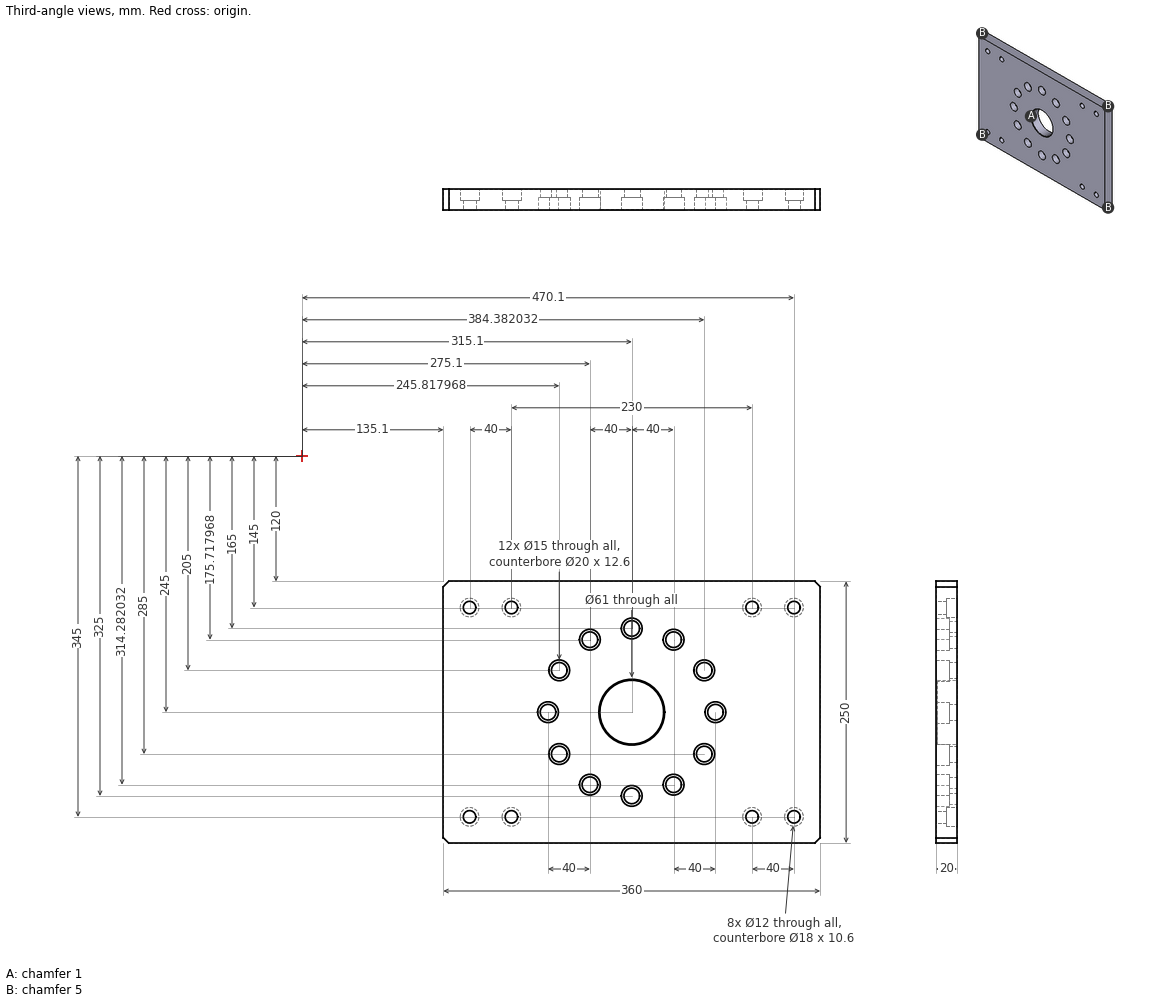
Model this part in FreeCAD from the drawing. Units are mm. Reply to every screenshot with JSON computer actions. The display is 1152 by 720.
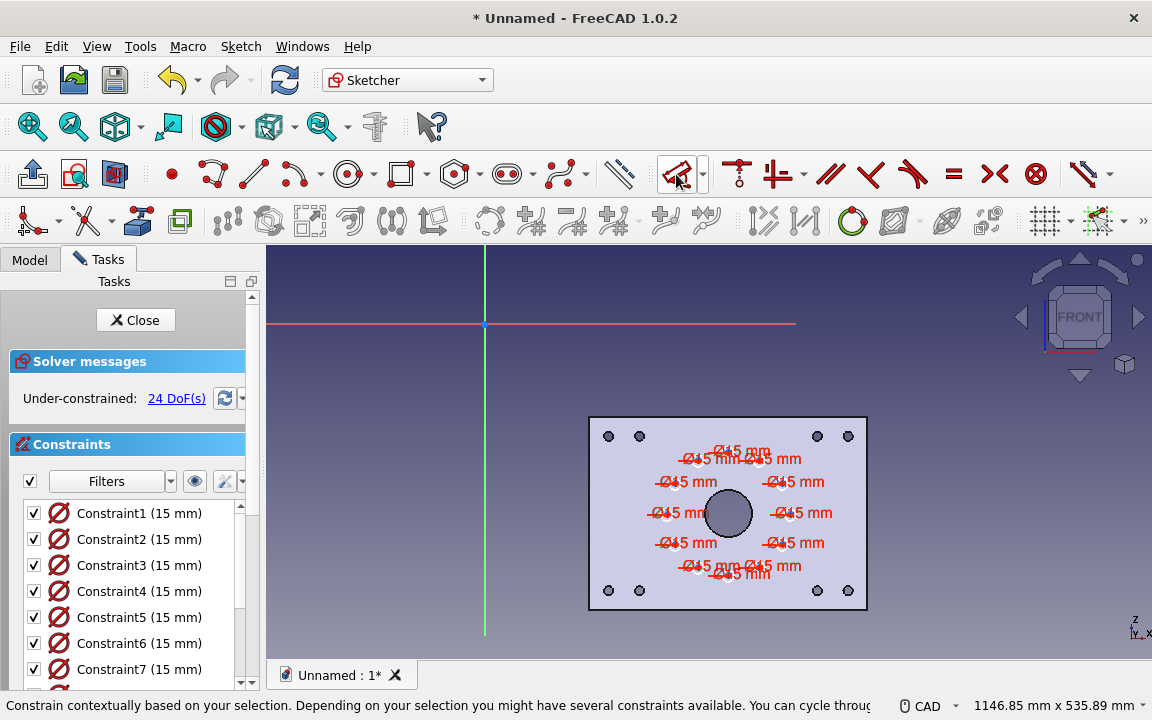
{"action": "left_click", "coordinate": [675, 484]}
{"action": "left_click", "coordinate": [451, 404]}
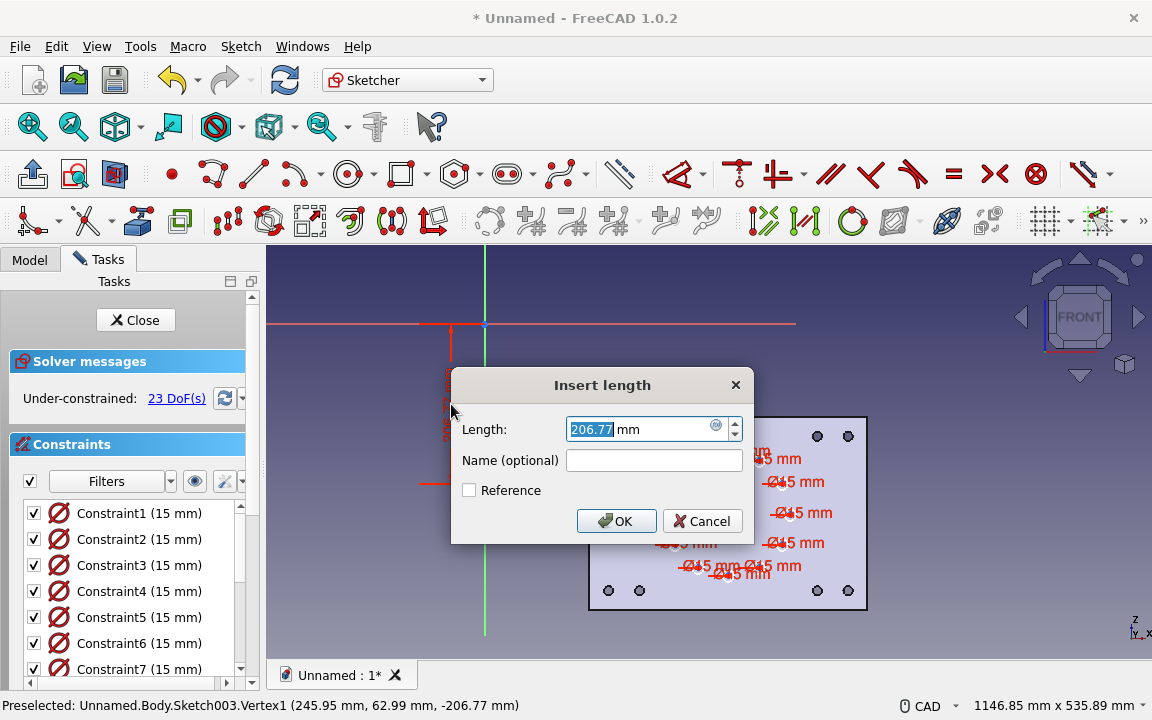
{"action": "type", "text": "205"}
{"action": "key", "text": "Return"}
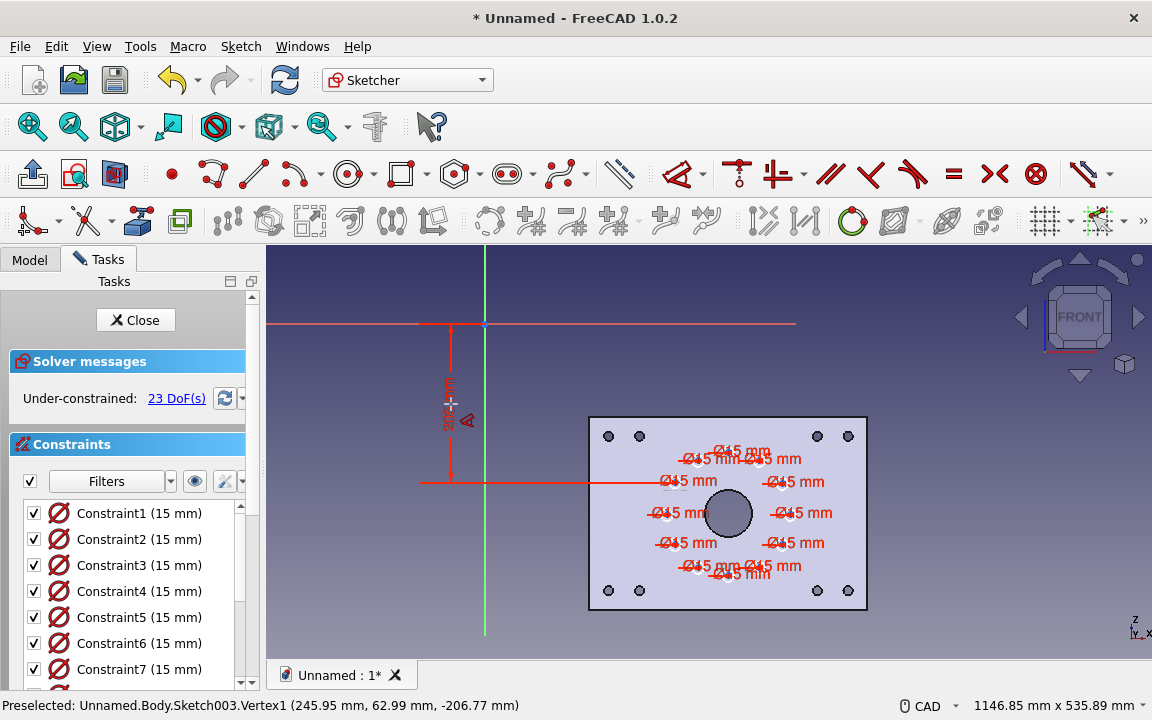
{"action": "left_click", "coordinate": [728, 453]}
{"action": "left_click", "coordinate": [451, 359]}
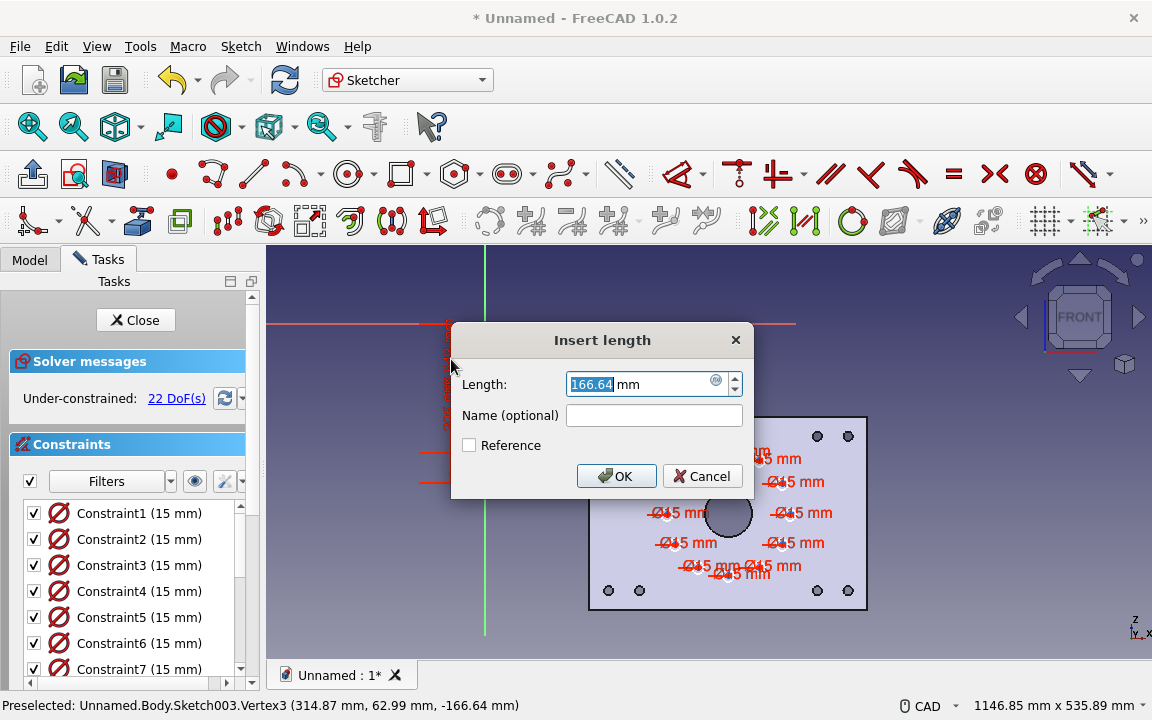
{"action": "type", "text": "165"}
{"action": "key", "text": "Return"}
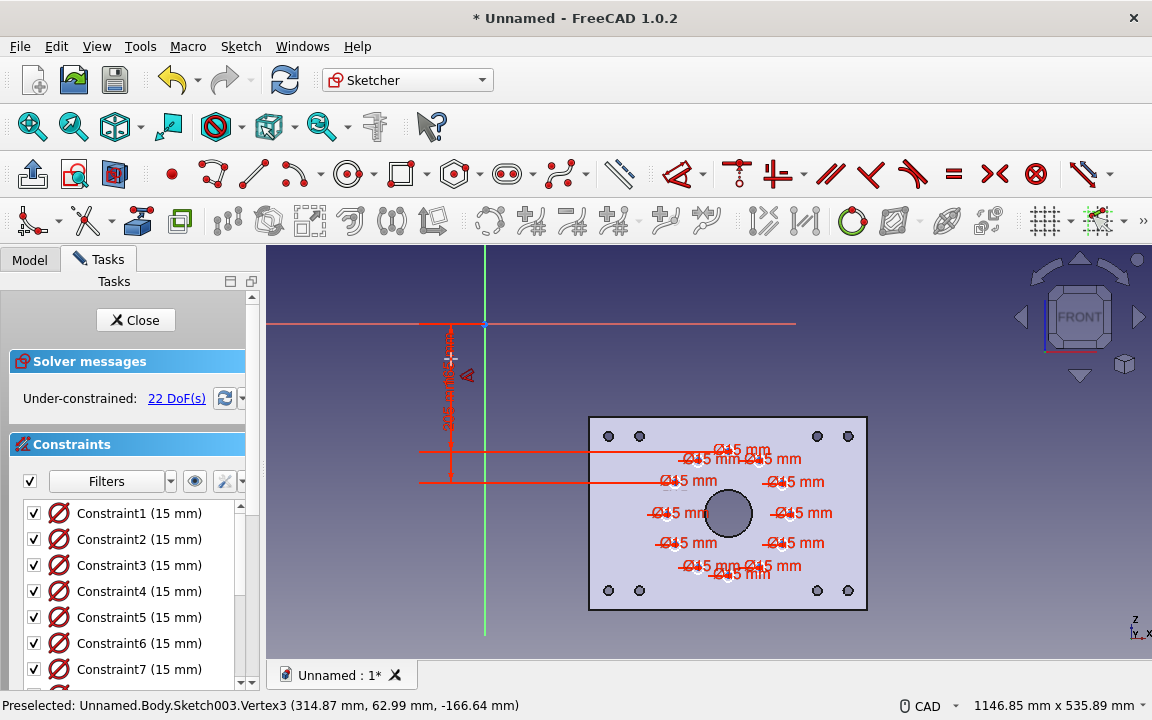
{"action": "left_click", "coordinate": [782, 484]}
{"action": "left_click", "coordinate": [451, 441]}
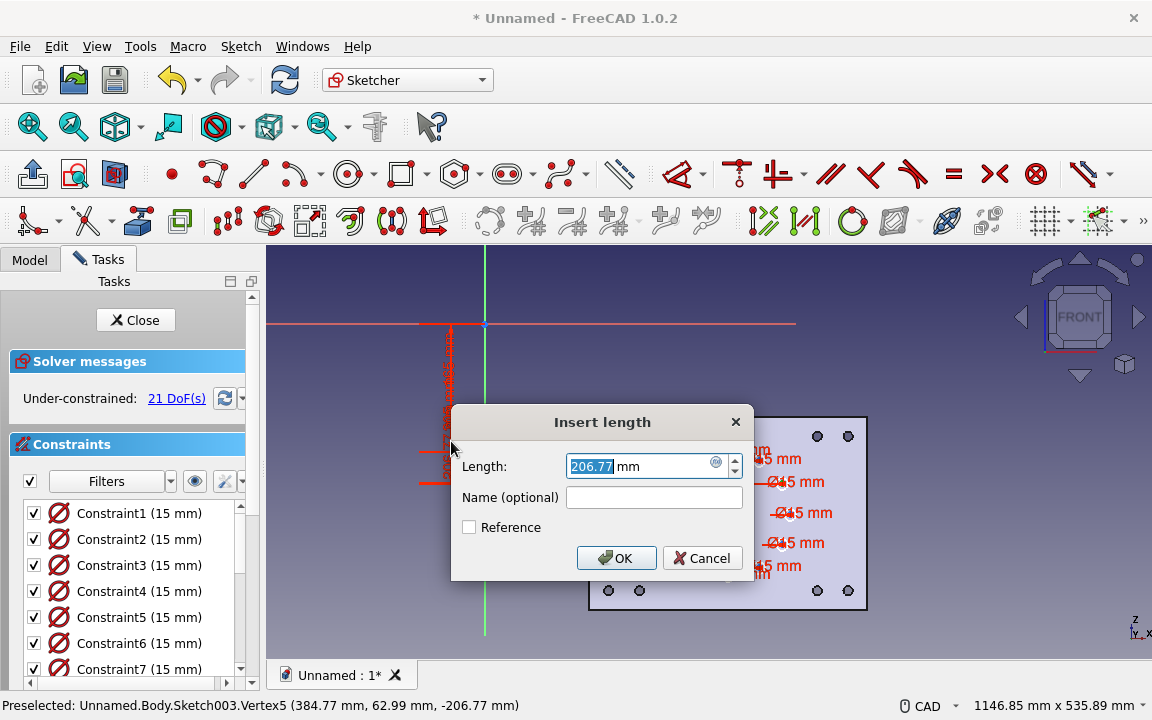
{"action": "type", "text": "205"}
{"action": "key", "text": "Return"}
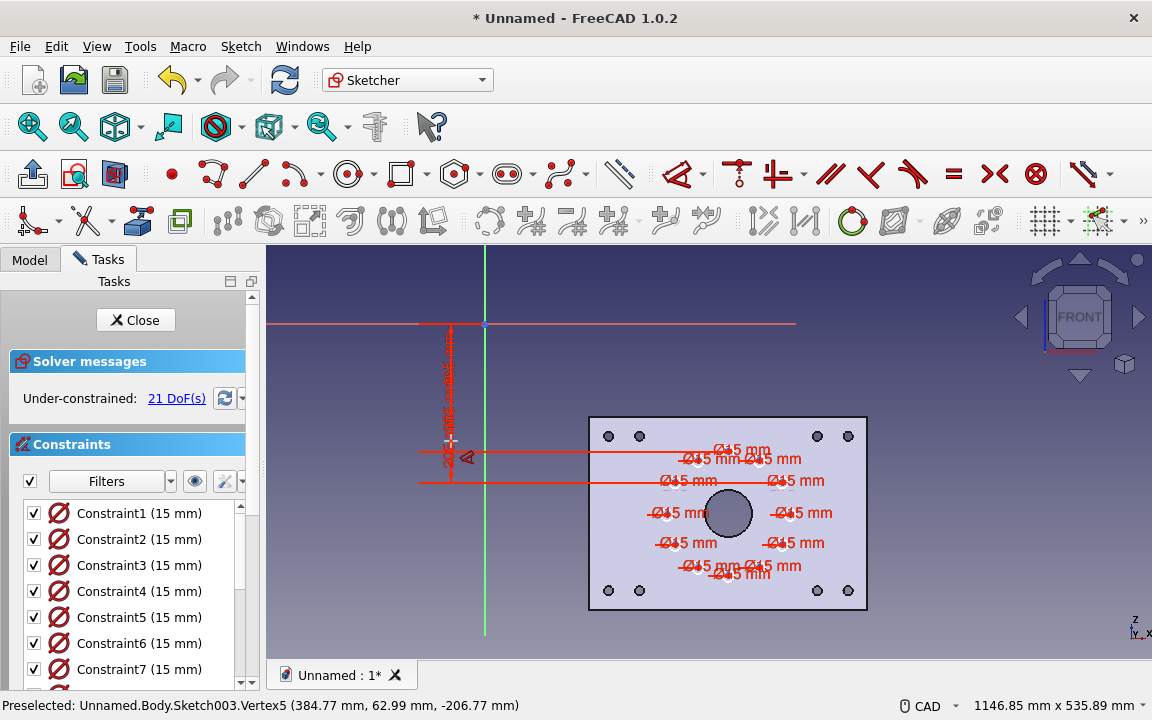
{"action": "left_click", "coordinate": [790, 515]}
{"action": "left_click", "coordinate": [451, 464]}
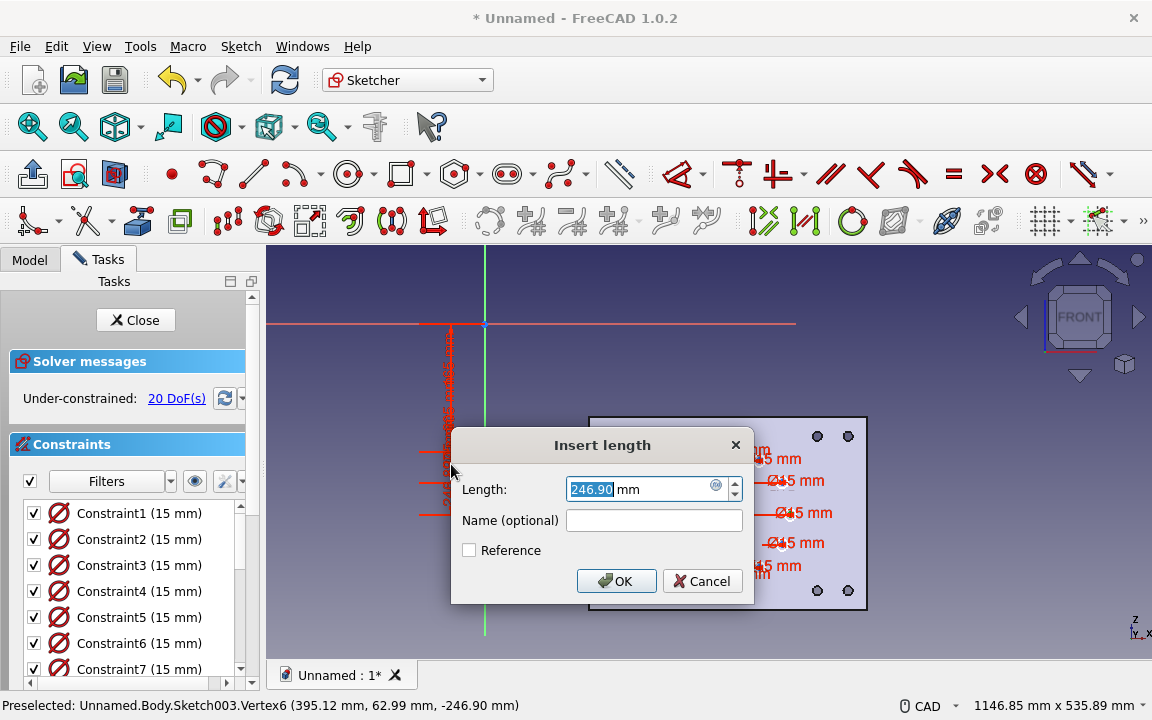
{"action": "type", "text": "245"}
{"action": "key", "text": "Return"}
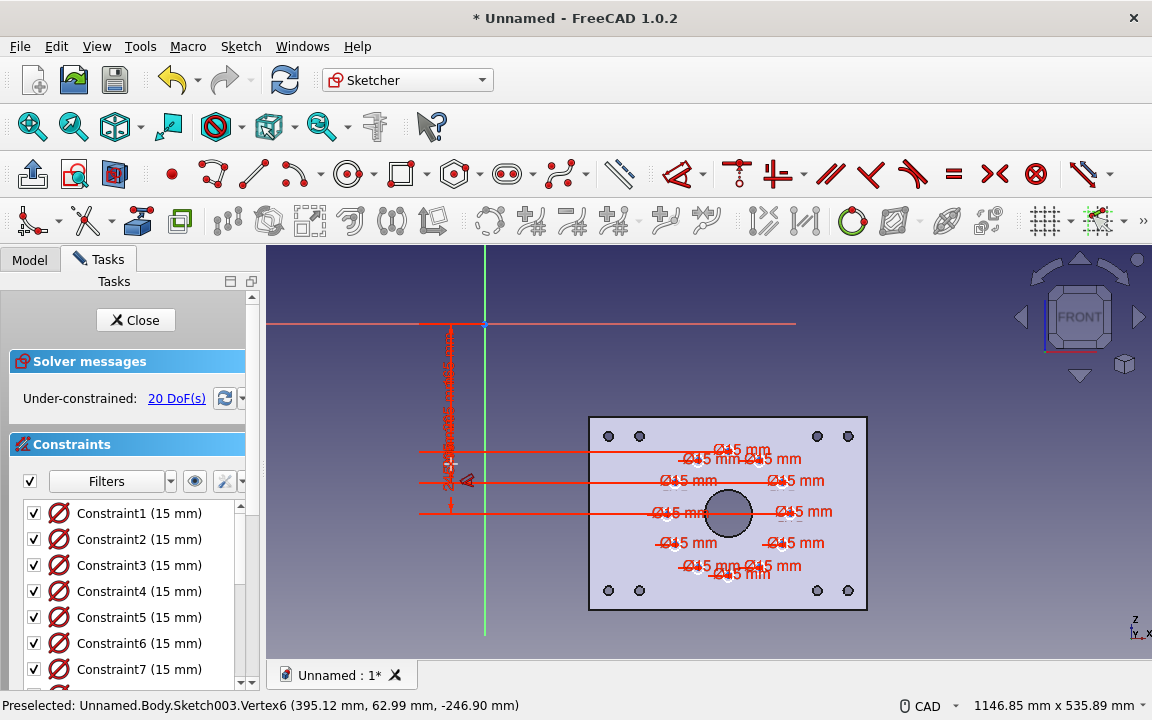
{"action": "left_click", "coordinate": [782, 545]}
{"action": "left_click", "coordinate": [451, 384]}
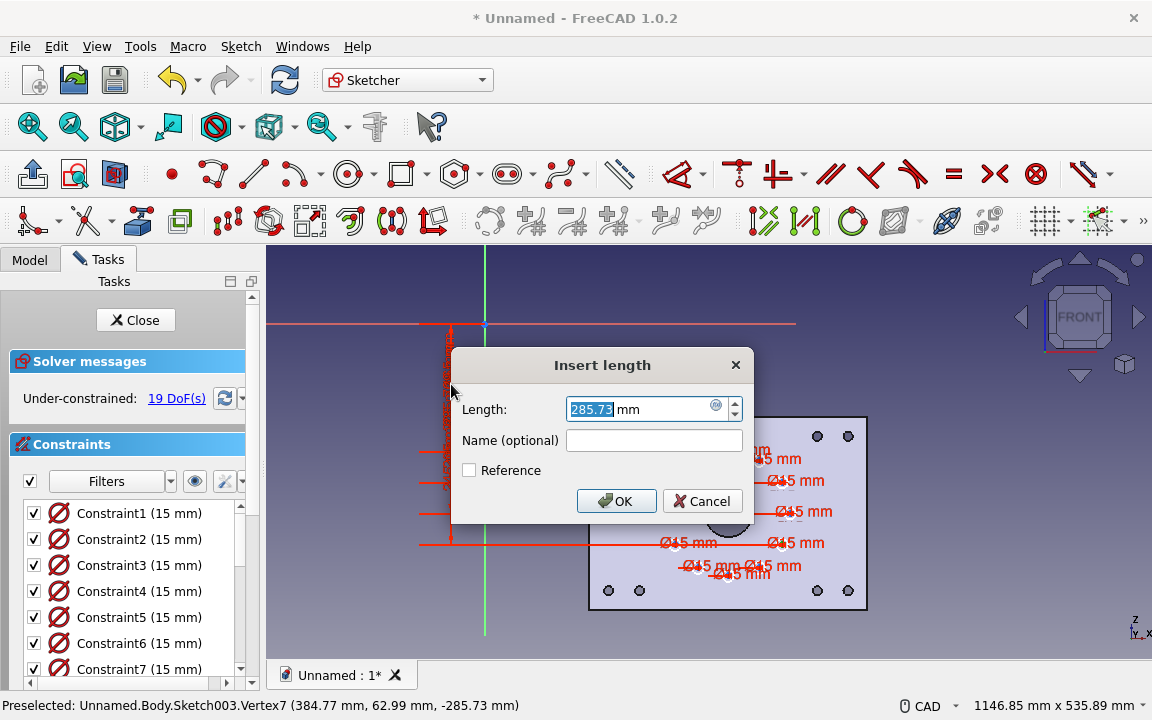
{"action": "type", "text": "285"}
{"action": "key", "text": "Return"}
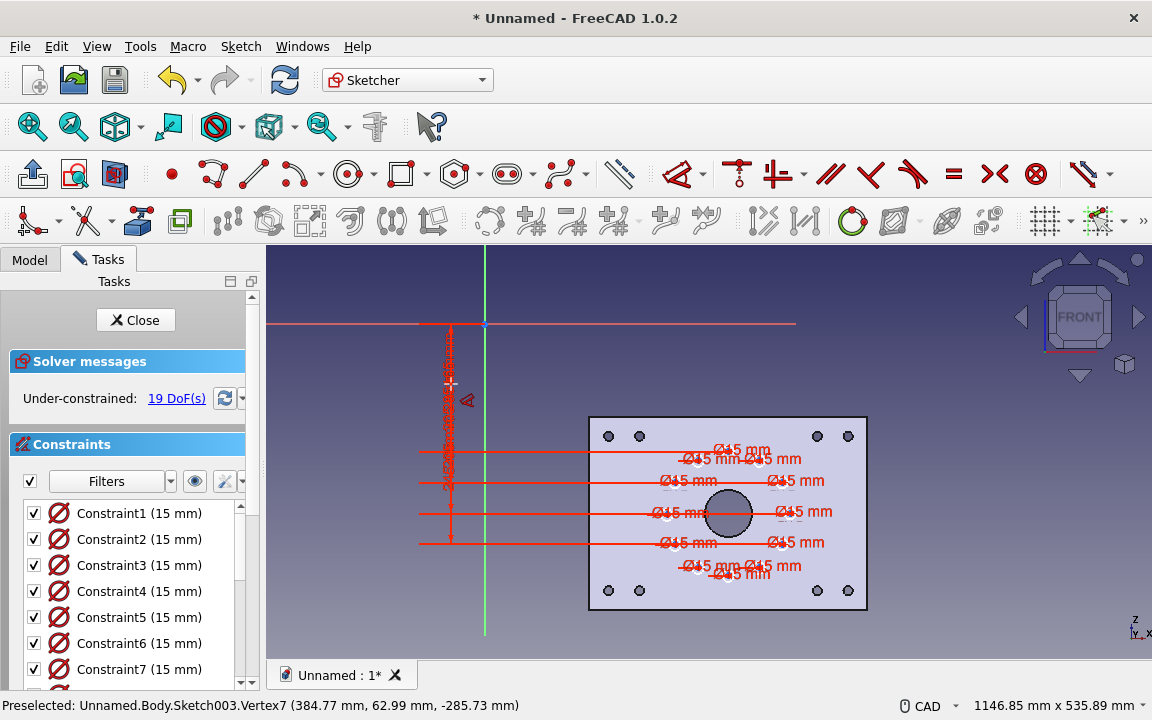
{"action": "left_click", "coordinate": [728, 576]}
{"action": "left_click", "coordinate": [451, 508]}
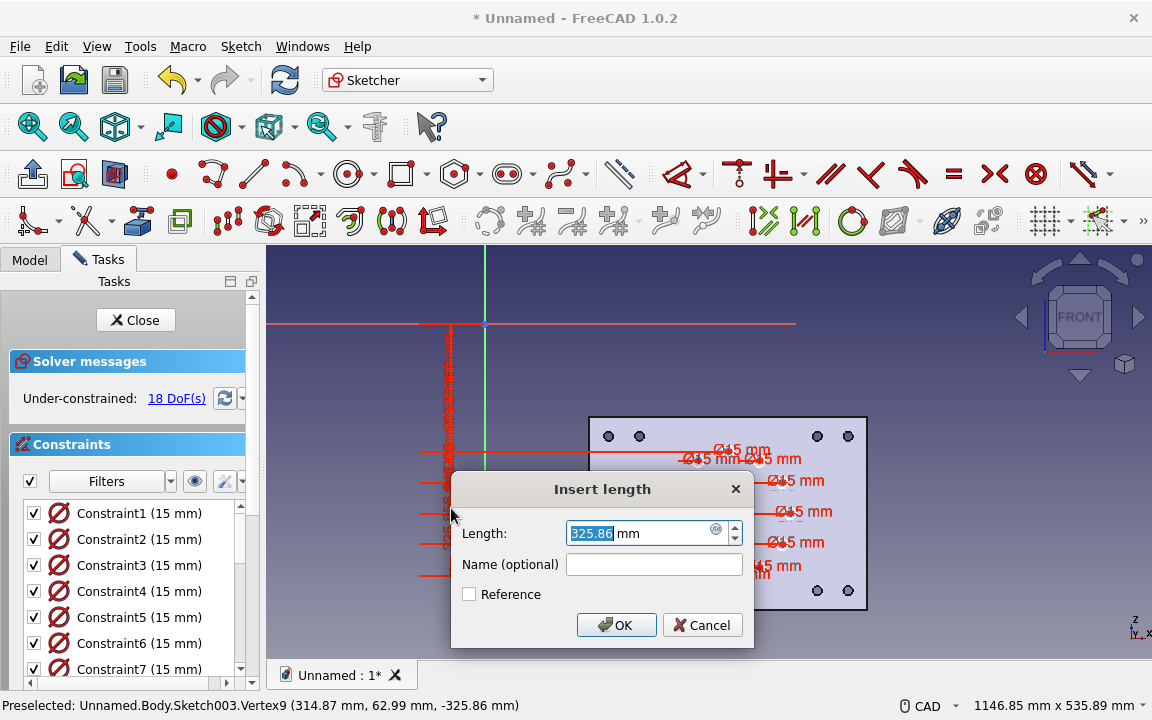
{"action": "type", "text": "325"}
{"action": "key", "text": "Return"}